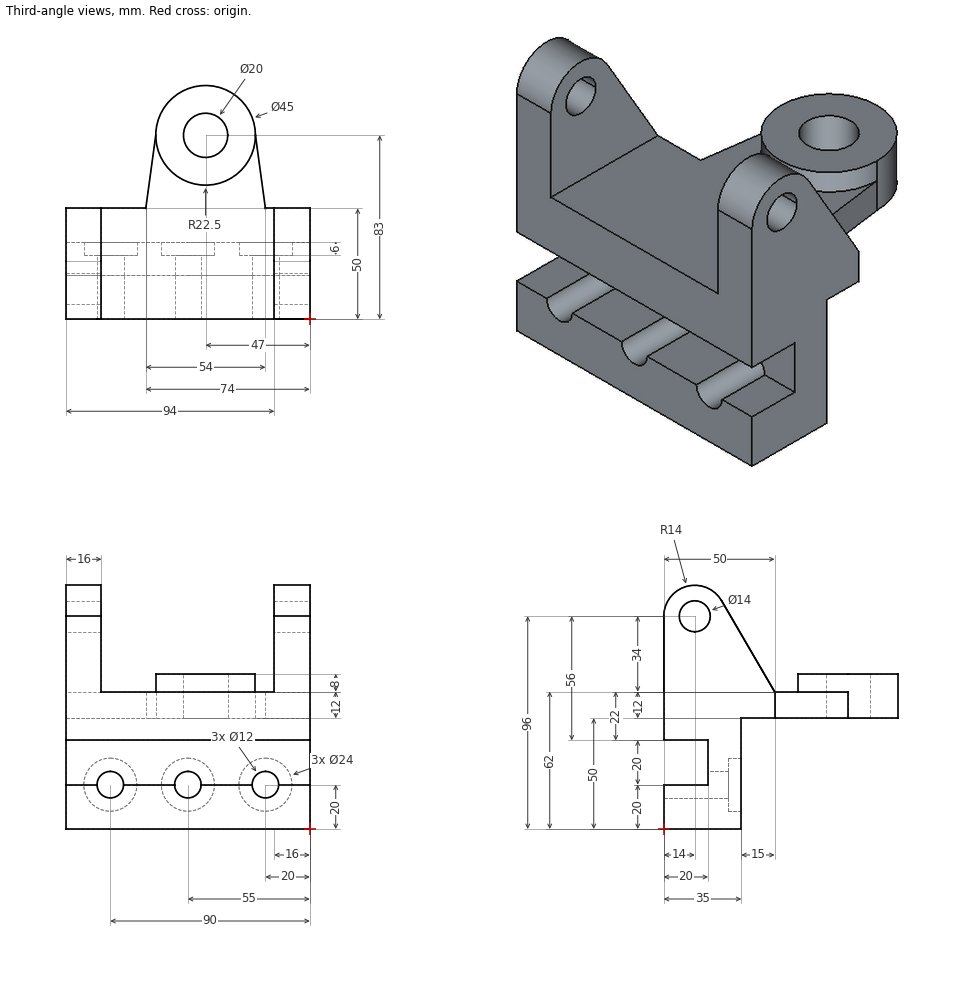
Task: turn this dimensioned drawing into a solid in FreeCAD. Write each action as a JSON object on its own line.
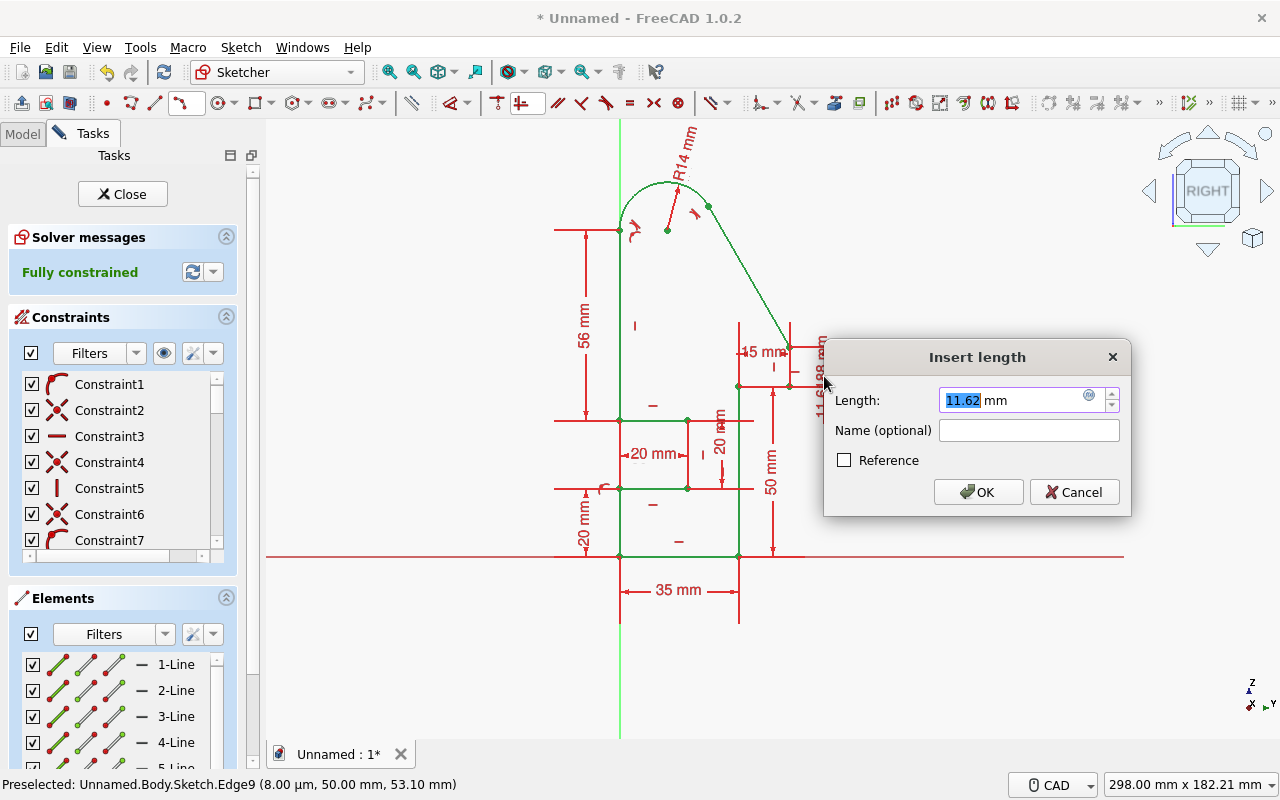
{"action": "type", "text": "12"}
{"action": "key", "text": "Return"}
{"action": "key", "text": "Escape"}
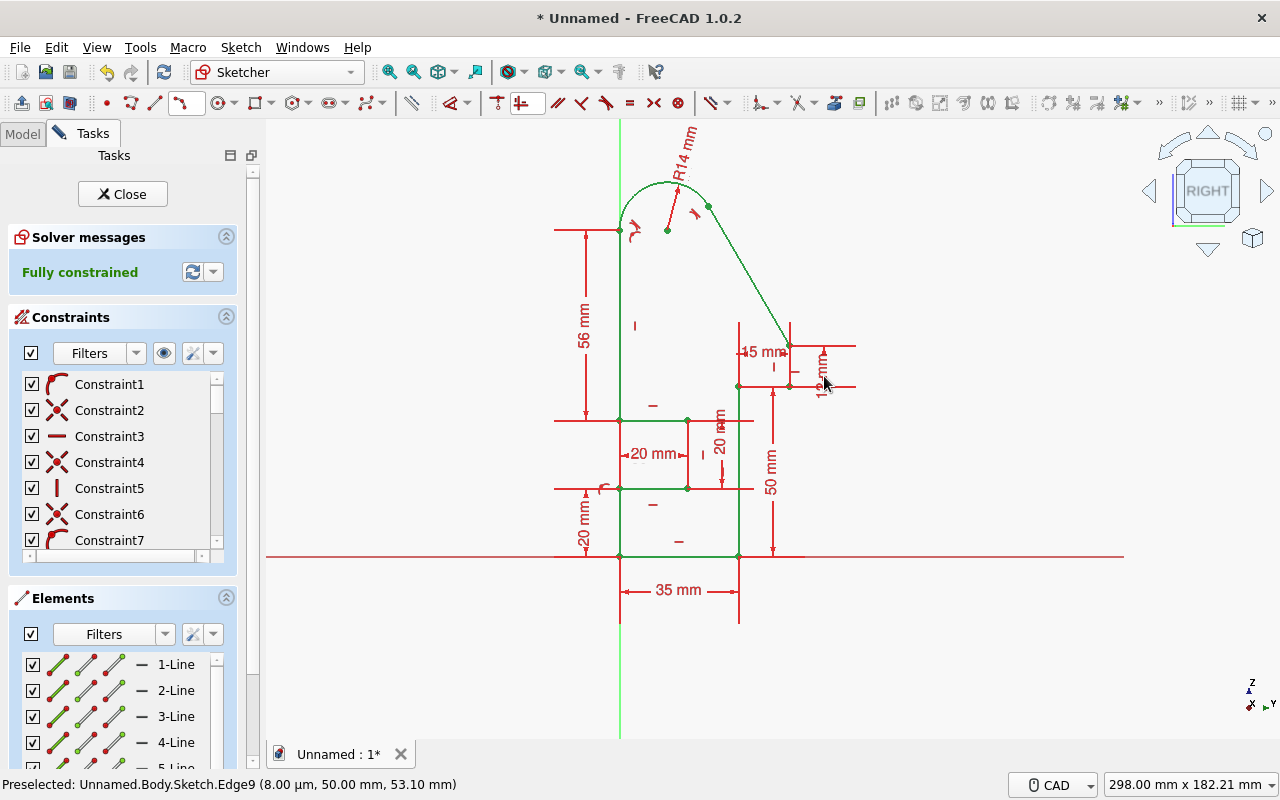
{"action": "left_click", "coordinate": [123, 194]}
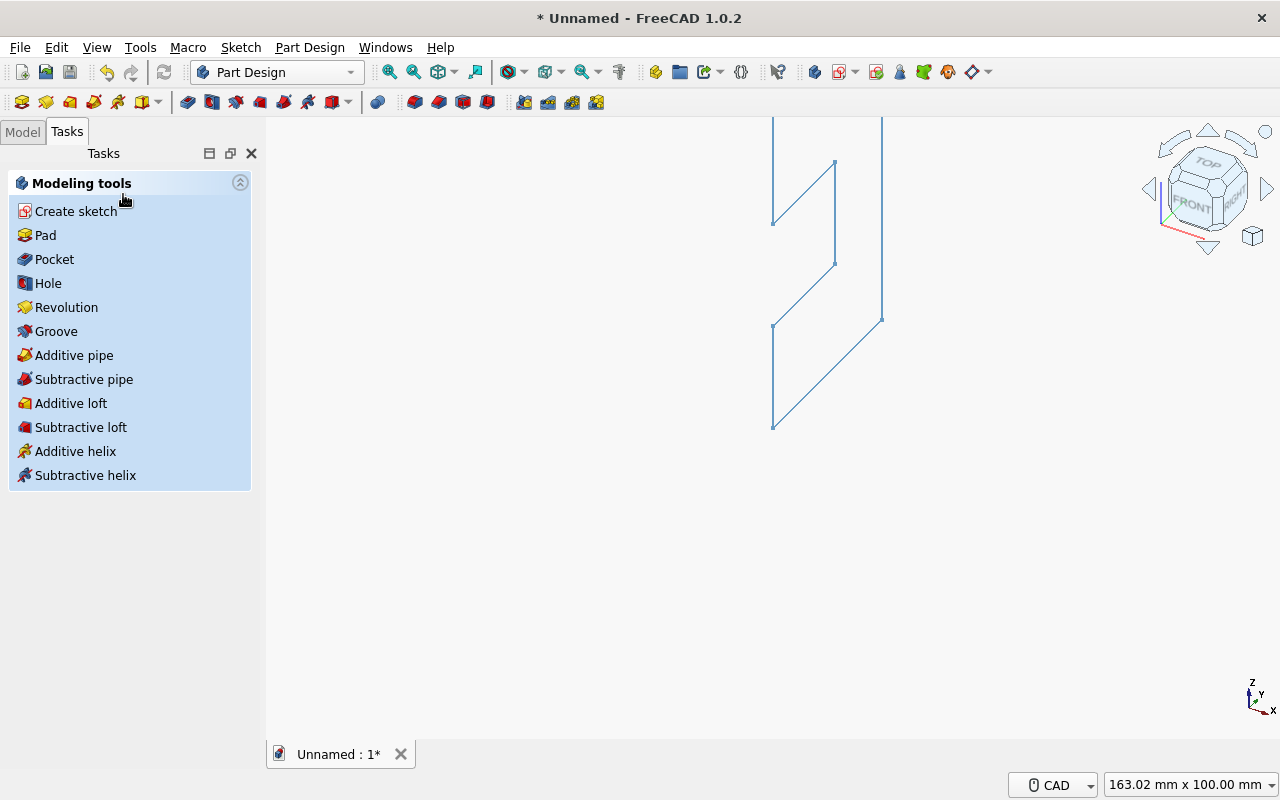
{"action": "left_click", "coordinate": [22, 102]}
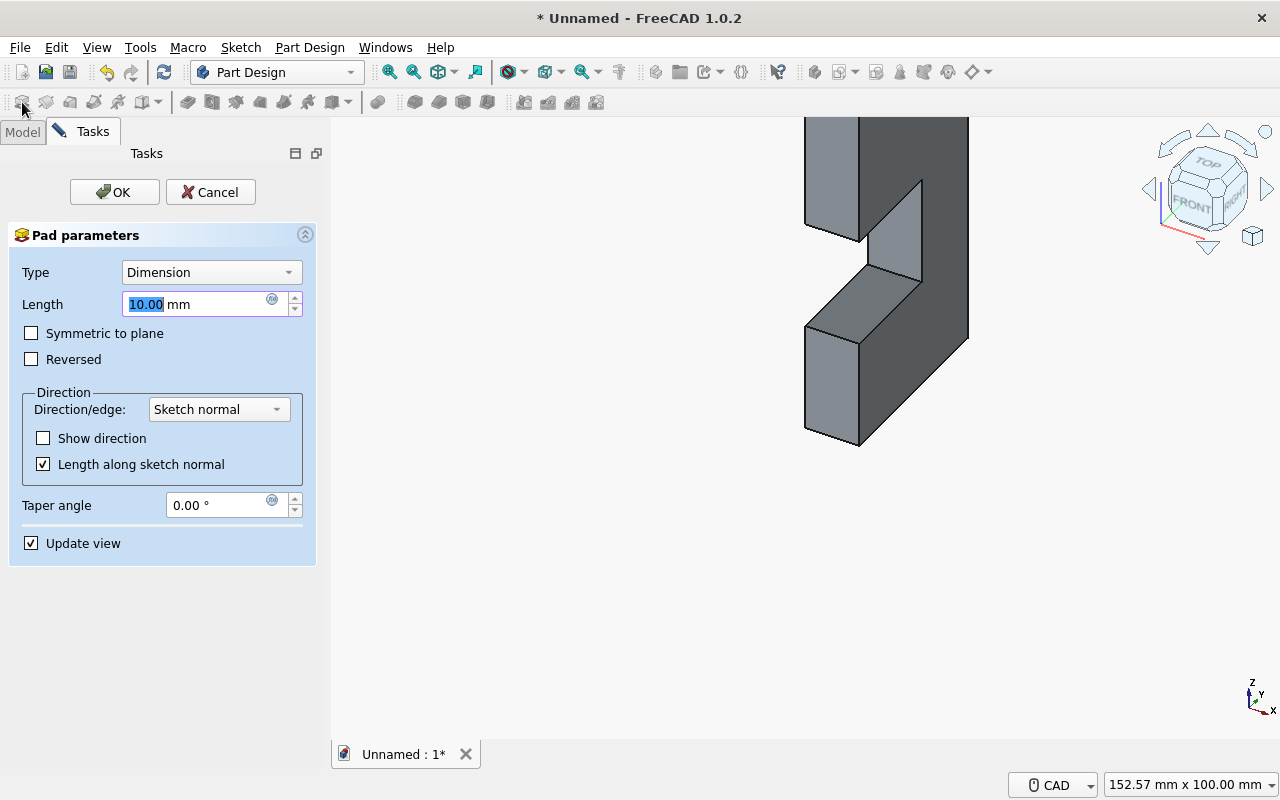
{"action": "type", "text": "16"}
{"action": "key", "text": "Tab"}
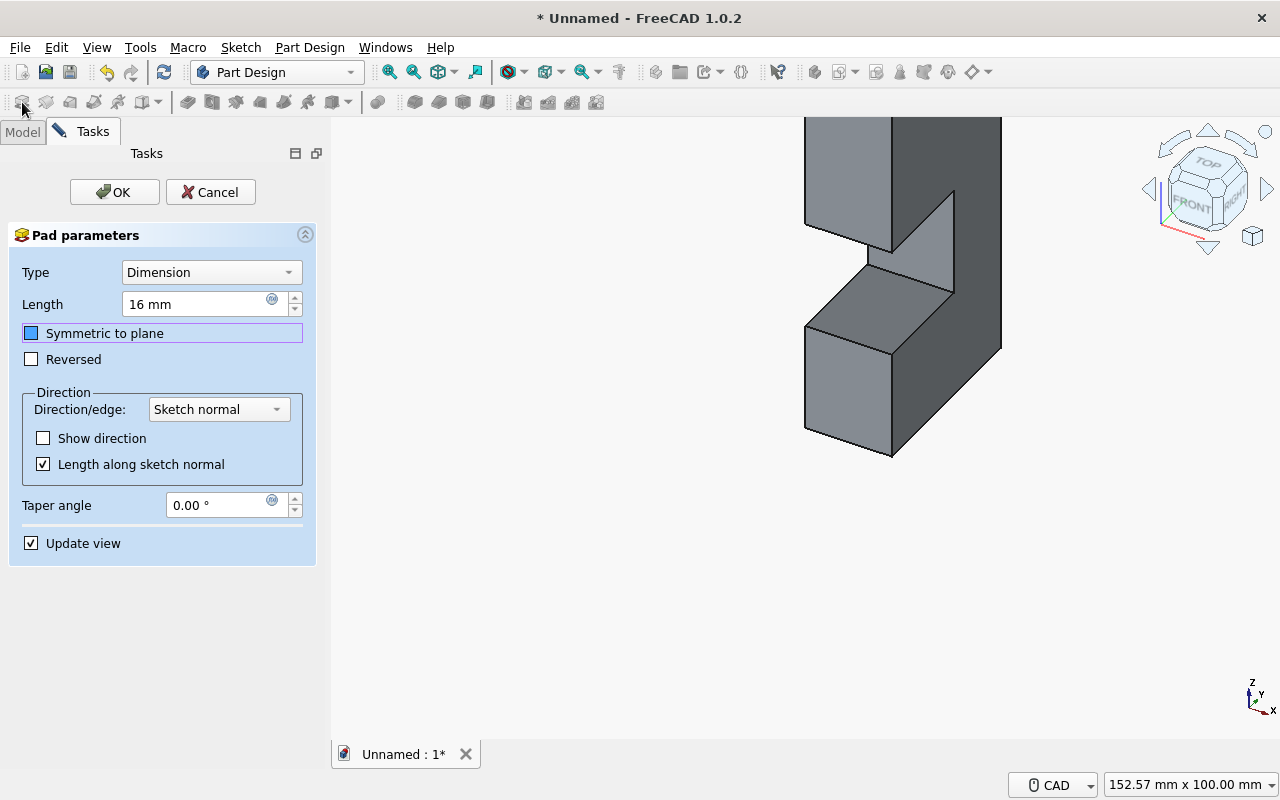
{"action": "left_click", "coordinate": [30, 359]}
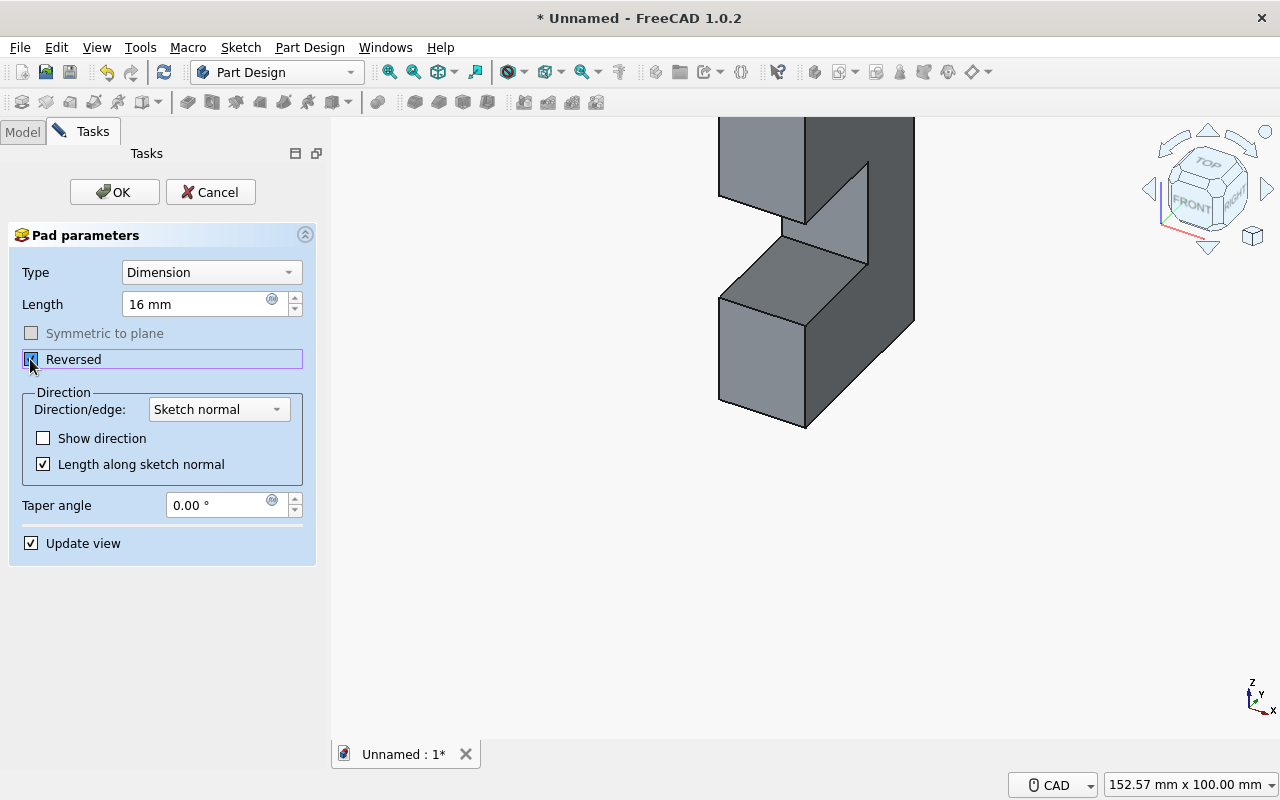
{"action": "left_click", "coordinate": [115, 192]}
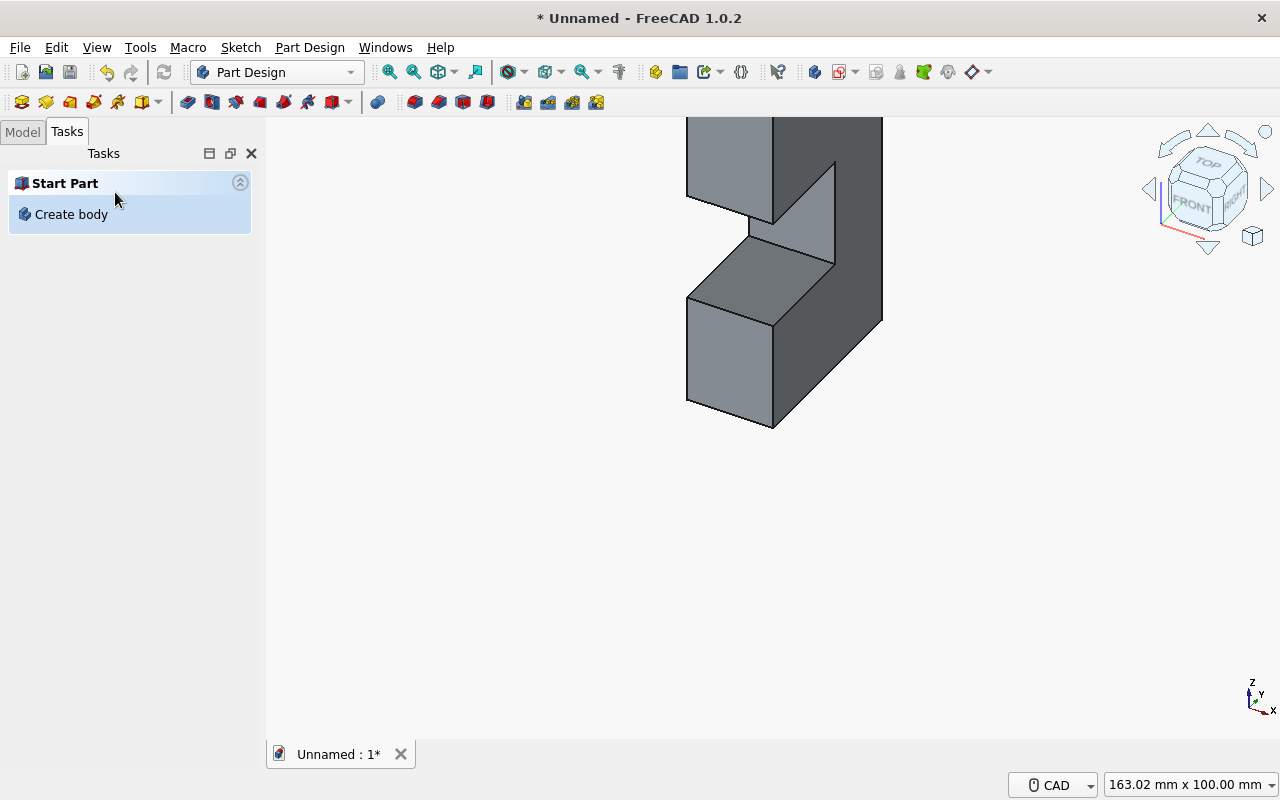
{"action": "key", "text": "v f"}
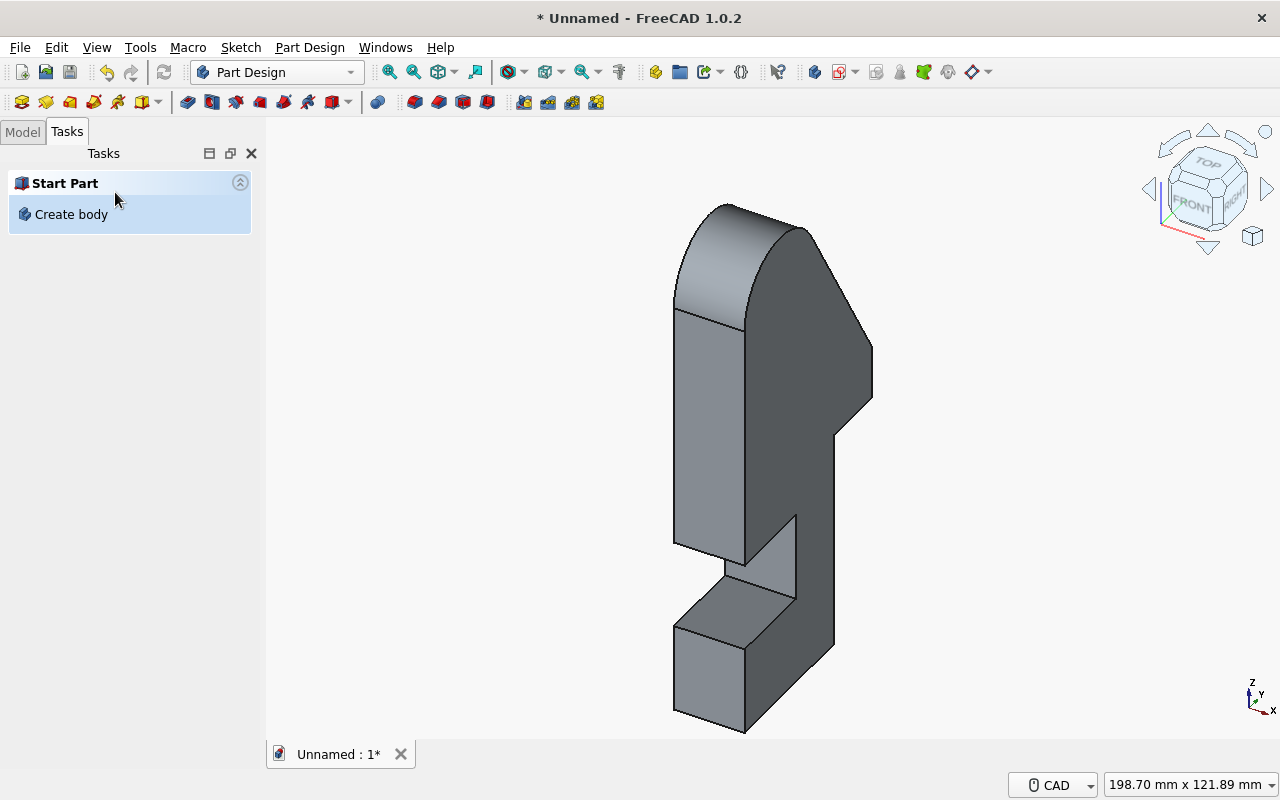
{"action": "key", "text": "6"}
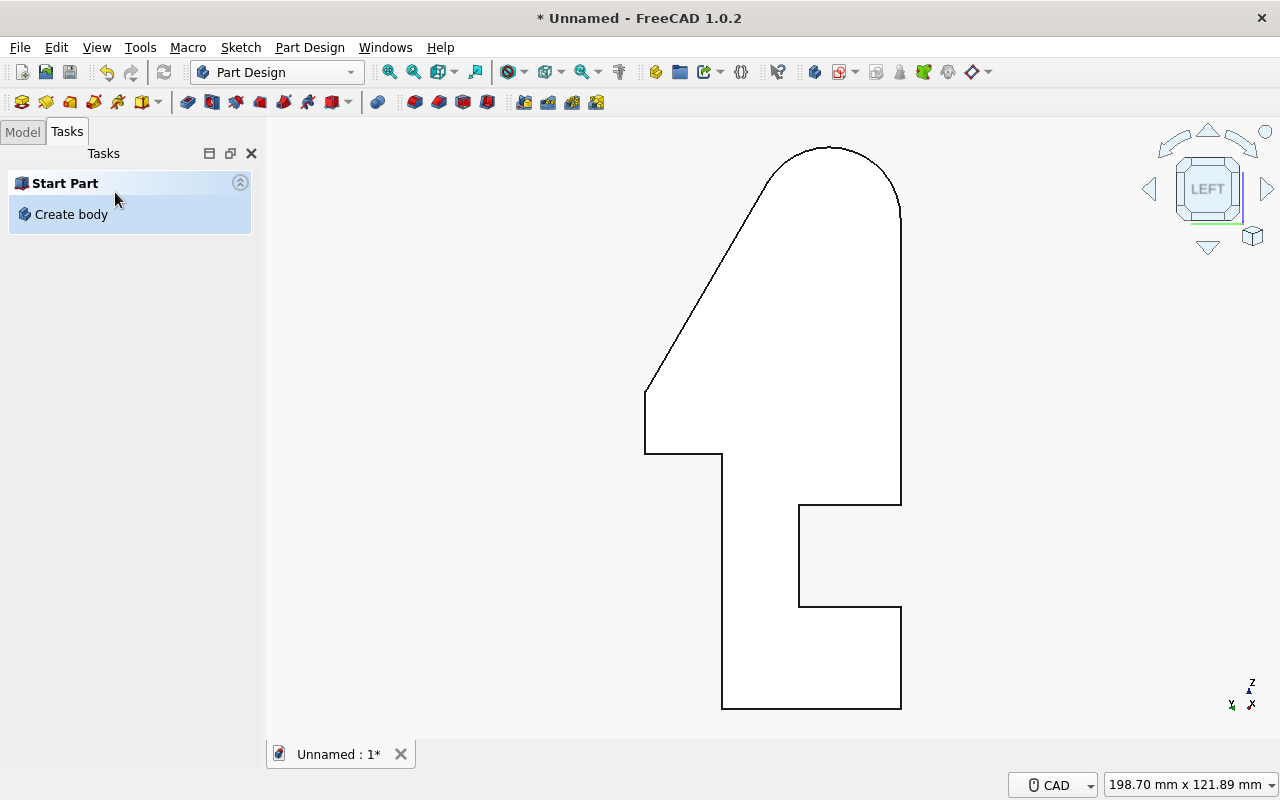
{"action": "left_click", "coordinate": [809, 347]}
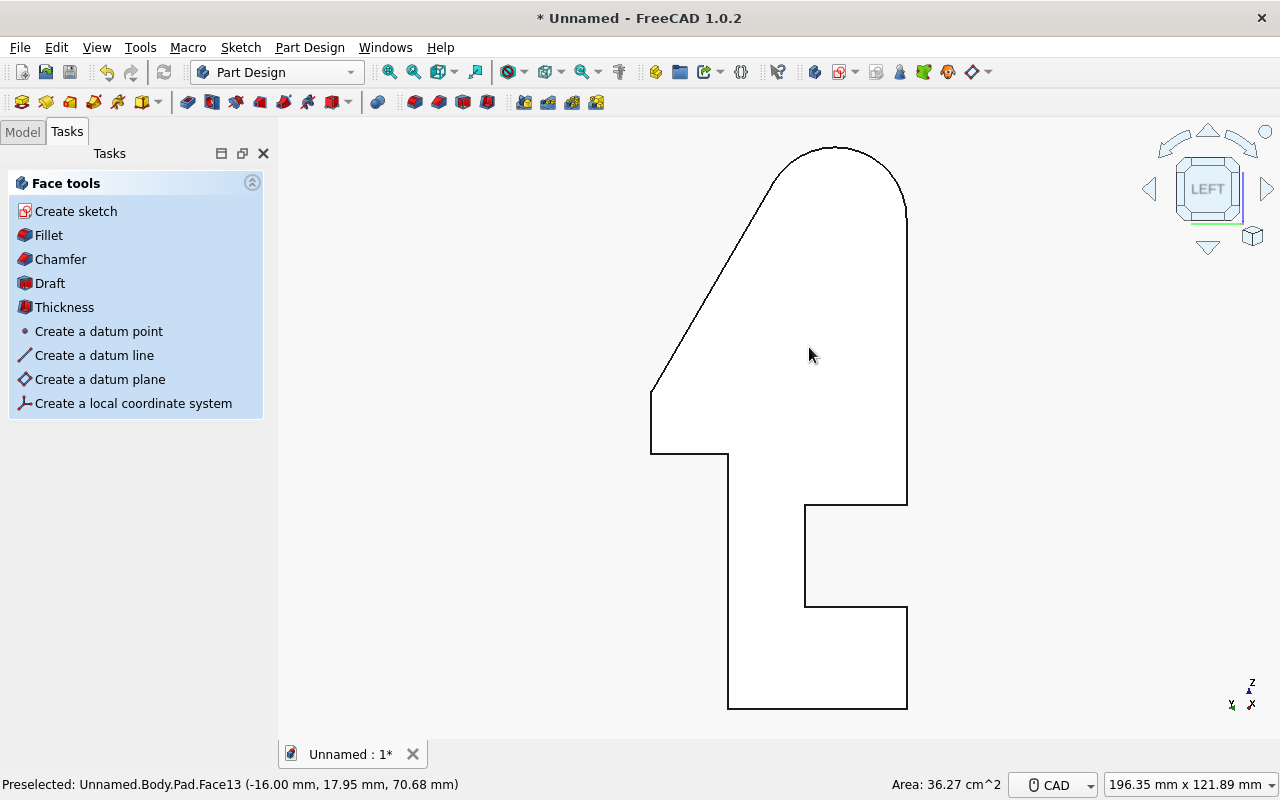
{"action": "left_click", "coordinate": [840, 72]}